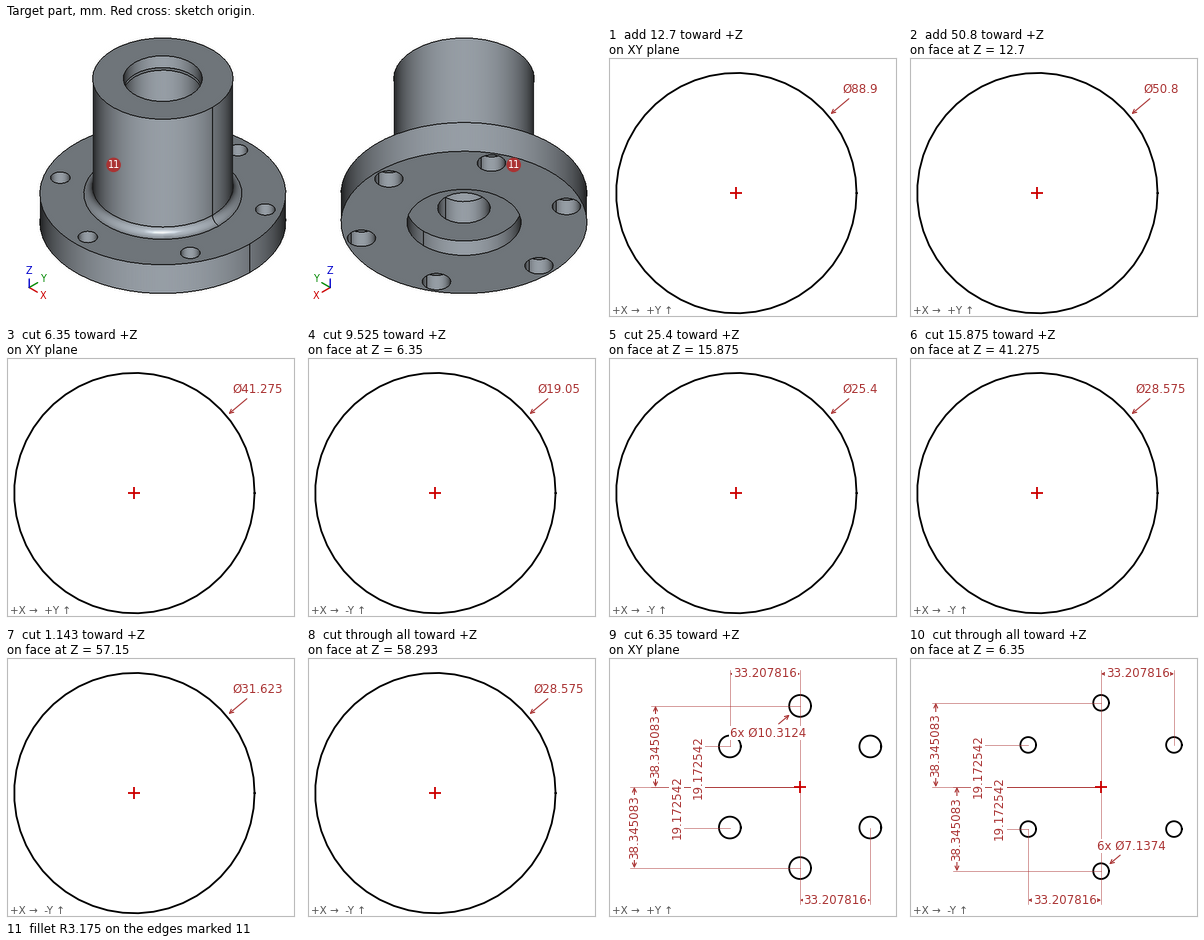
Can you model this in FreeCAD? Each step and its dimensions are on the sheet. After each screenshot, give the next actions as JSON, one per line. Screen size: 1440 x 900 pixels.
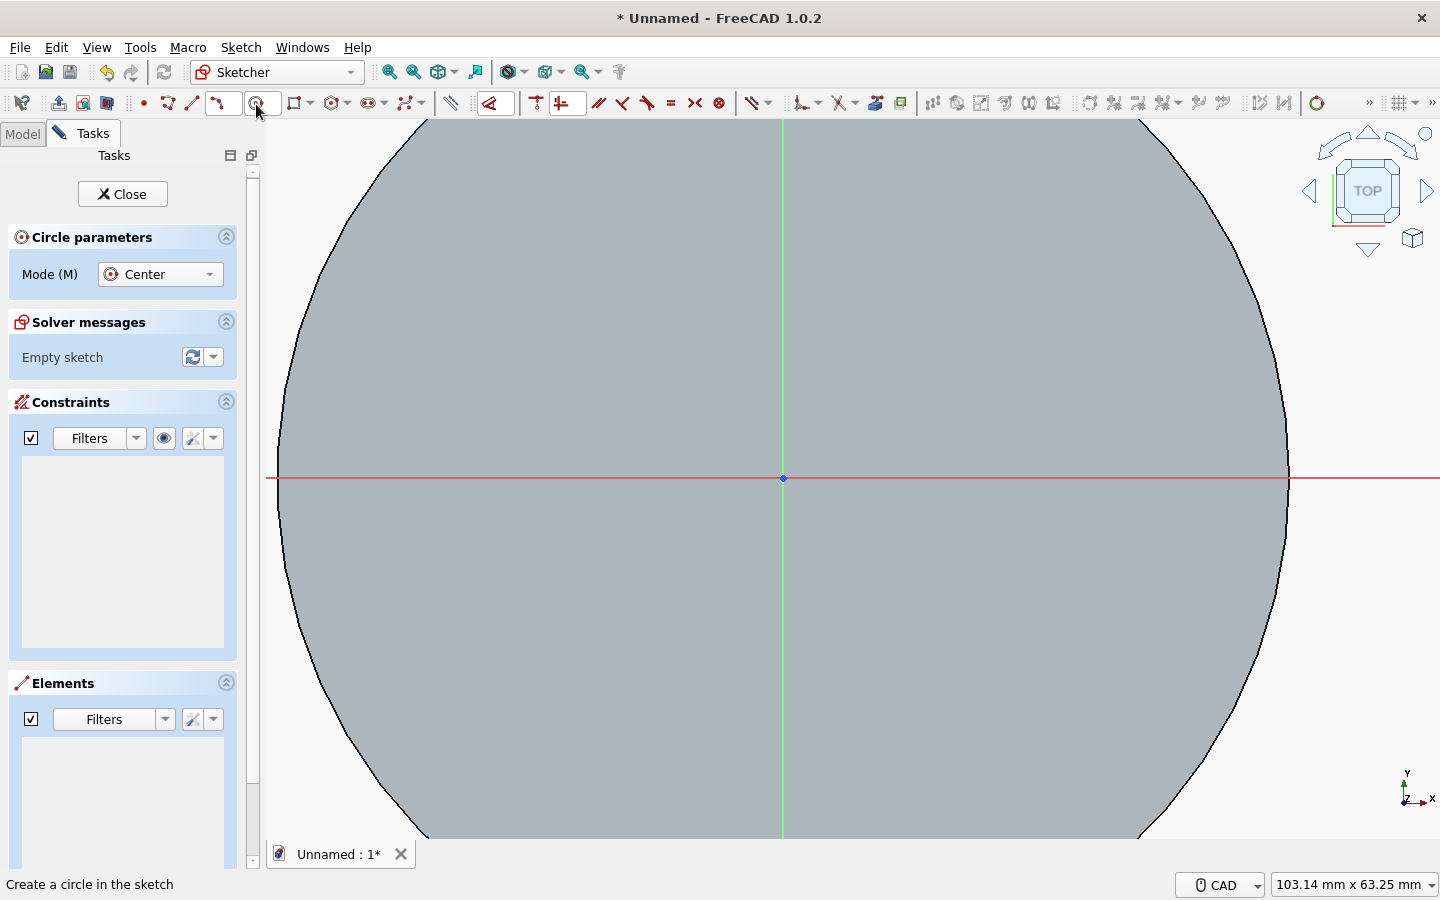
{"action": "left_click", "coordinate": [783, 478]}
{"action": "mouse_move", "coordinate": [949, 312]}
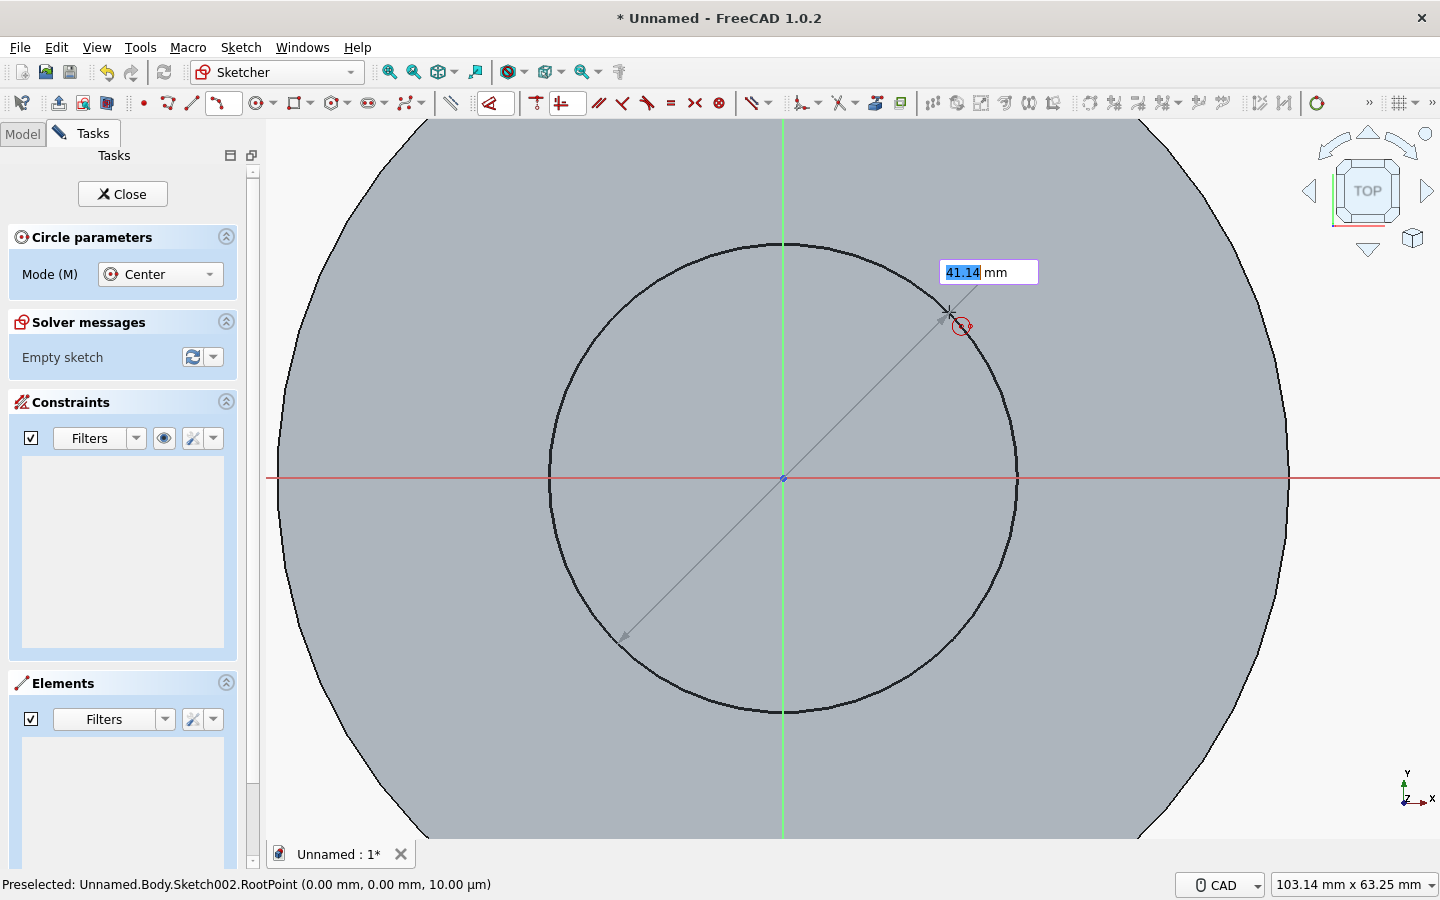
{"action": "type", "text": "41.275"}
{"action": "key", "text": "Return"}
{"action": "key", "text": "Escape"}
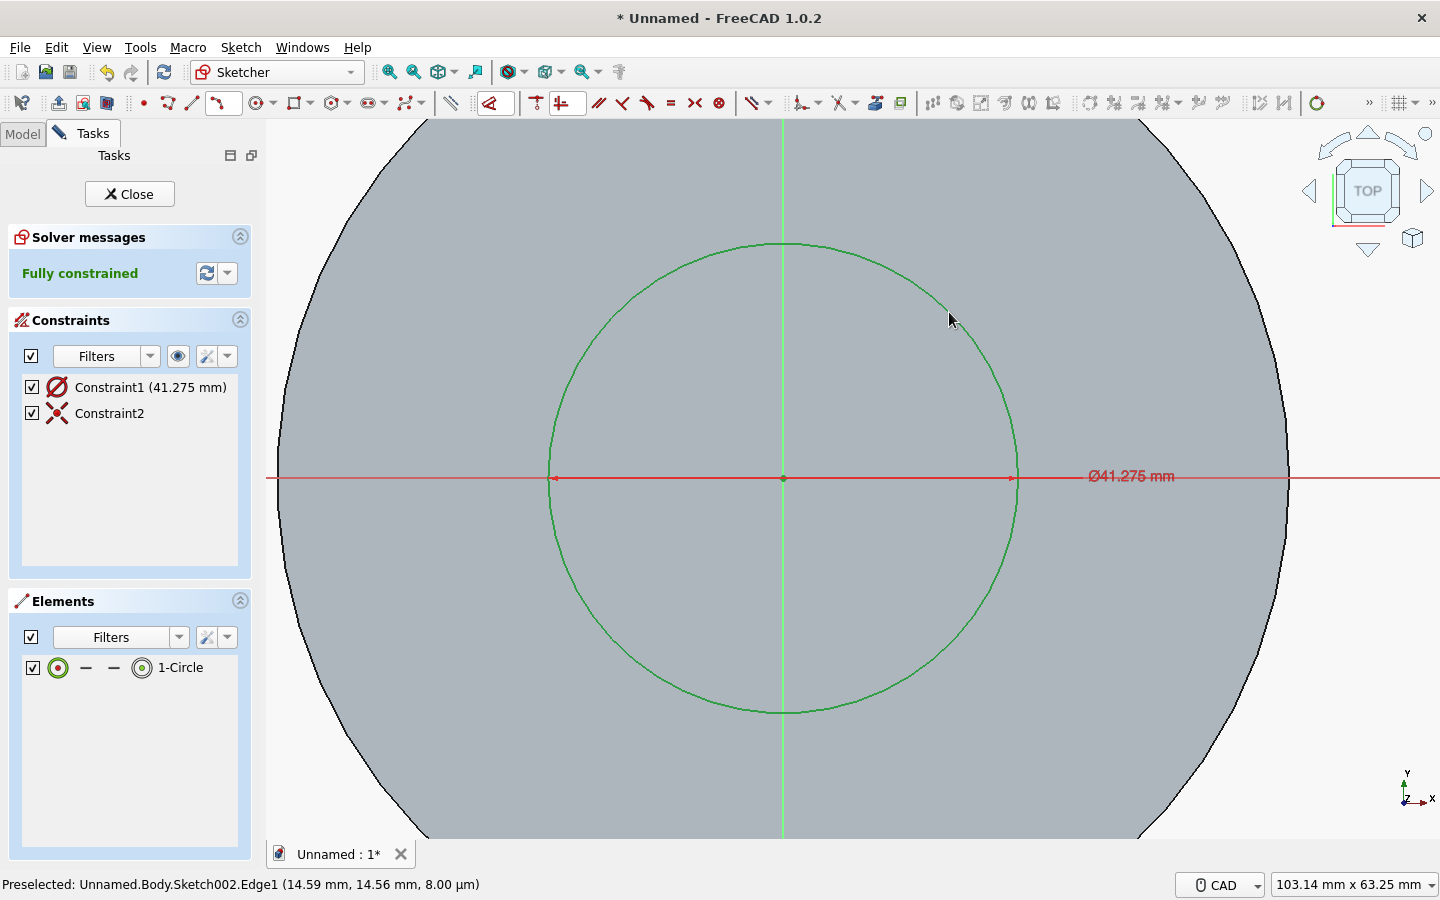
{"action": "left_click", "coordinate": [130, 194]}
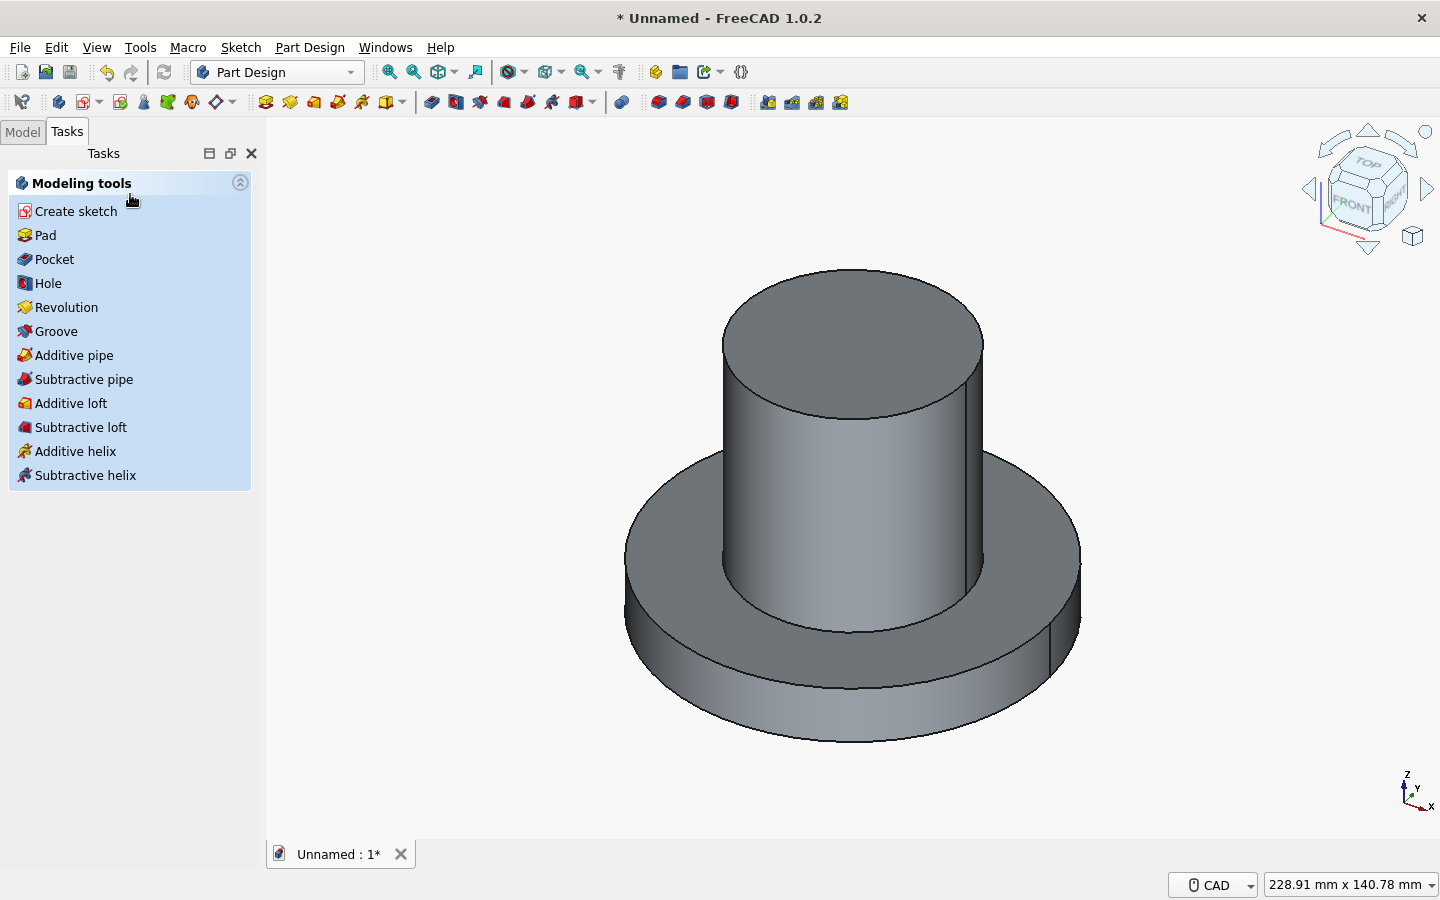
{"action": "left_click", "coordinate": [432, 102]}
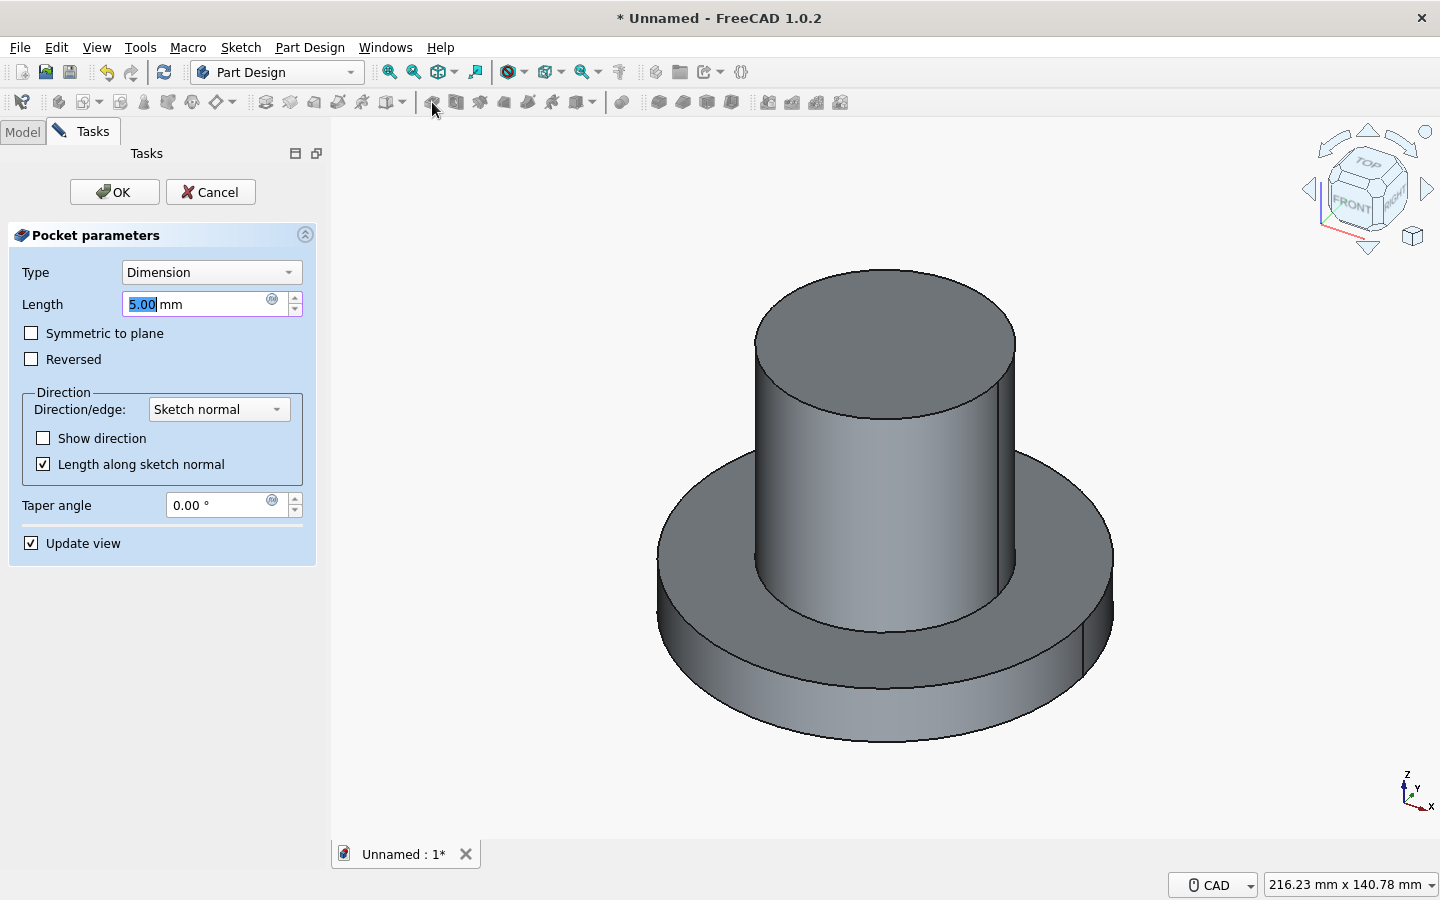
{"action": "type", "text": "6.35"}
{"action": "key", "text": "Tab"}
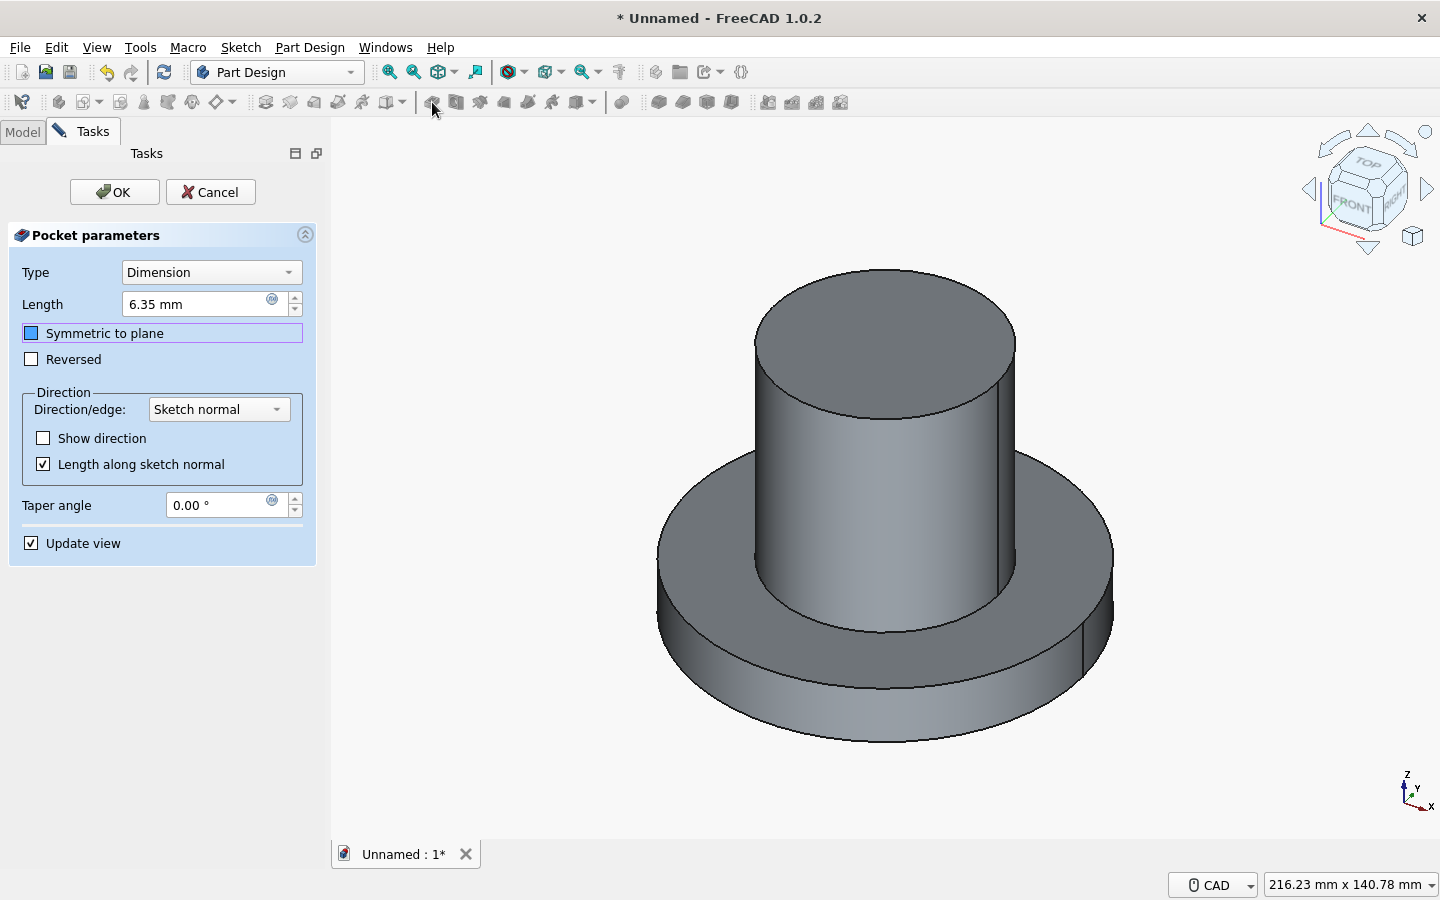
{"action": "left_click", "coordinate": [30, 359]}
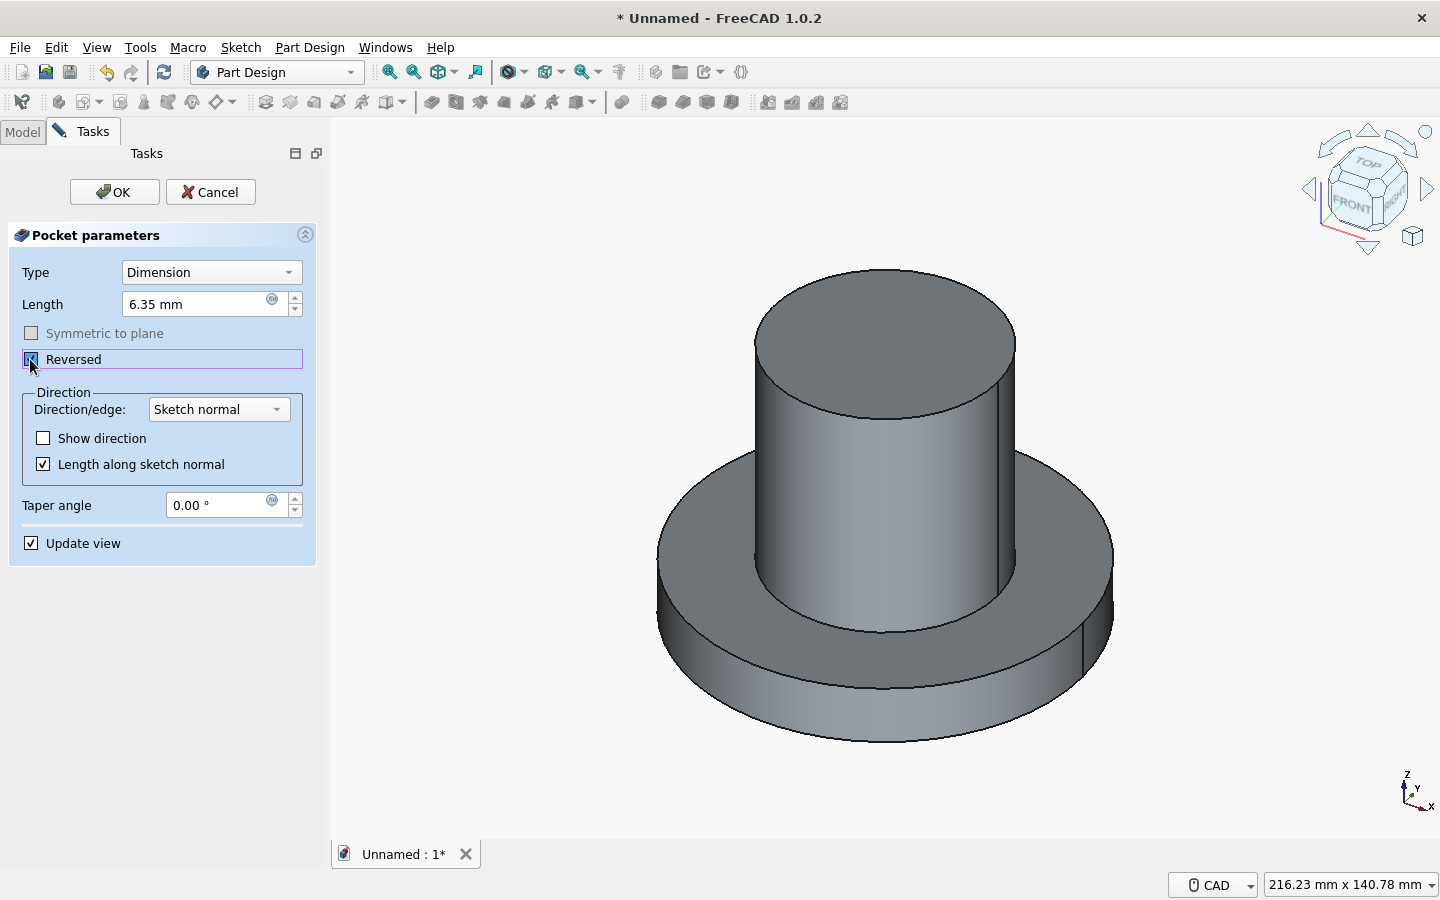
{"action": "left_click", "coordinate": [115, 192]}